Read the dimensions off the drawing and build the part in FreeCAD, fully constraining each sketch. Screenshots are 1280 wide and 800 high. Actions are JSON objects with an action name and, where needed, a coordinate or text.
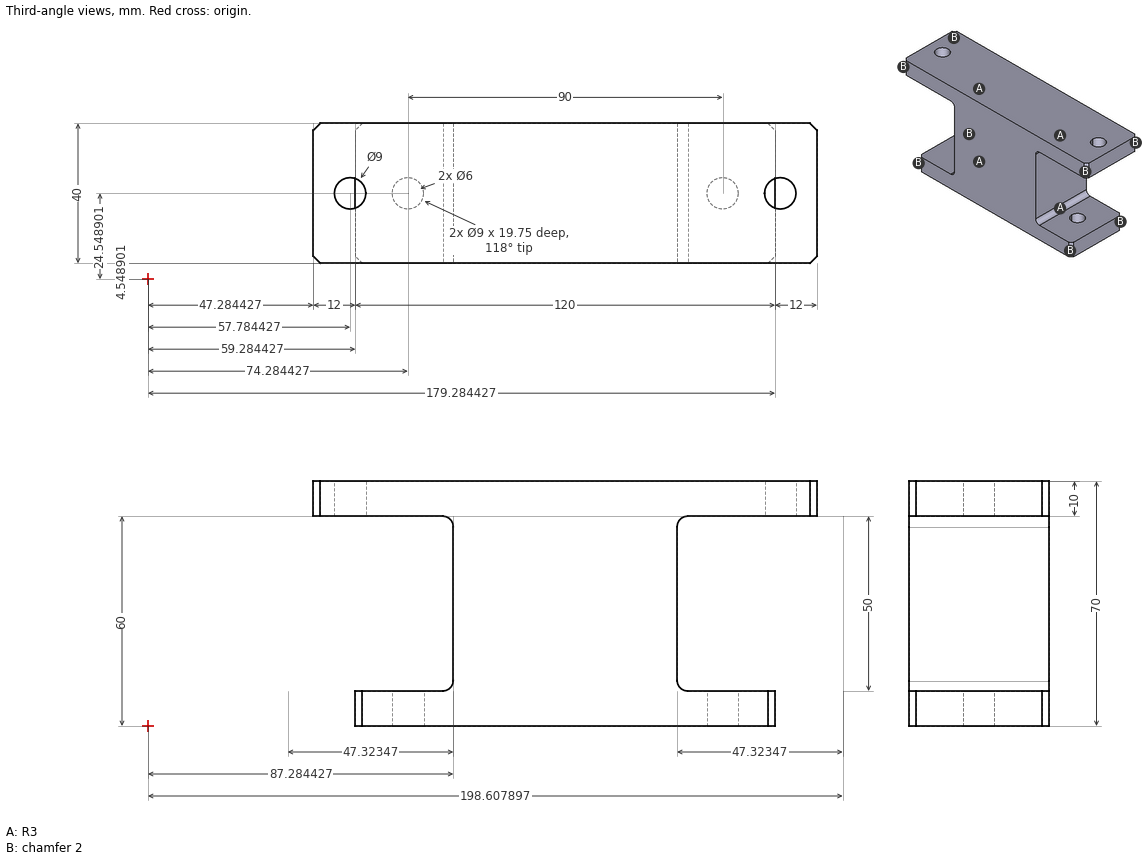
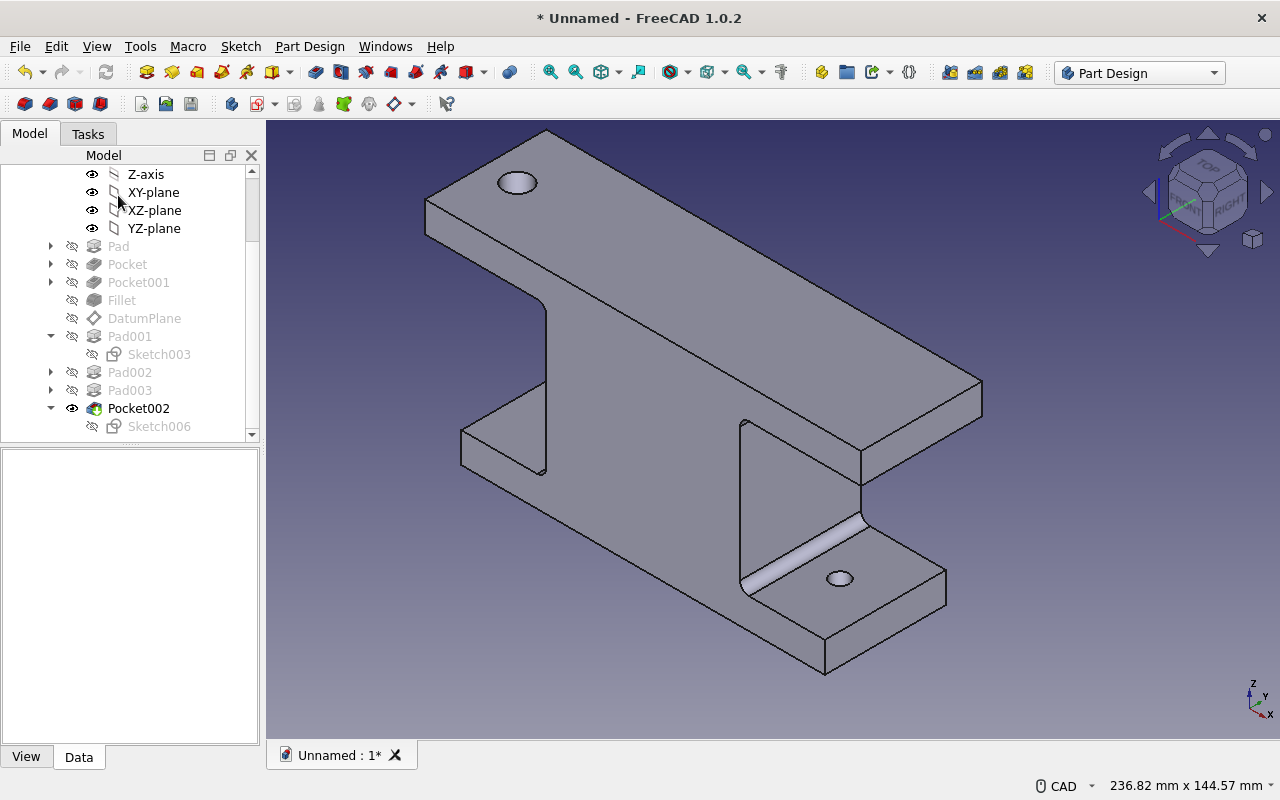
{"action": "scroll", "coordinate": [161, 296], "scroll_direction": "down", "scroll_amount": 3}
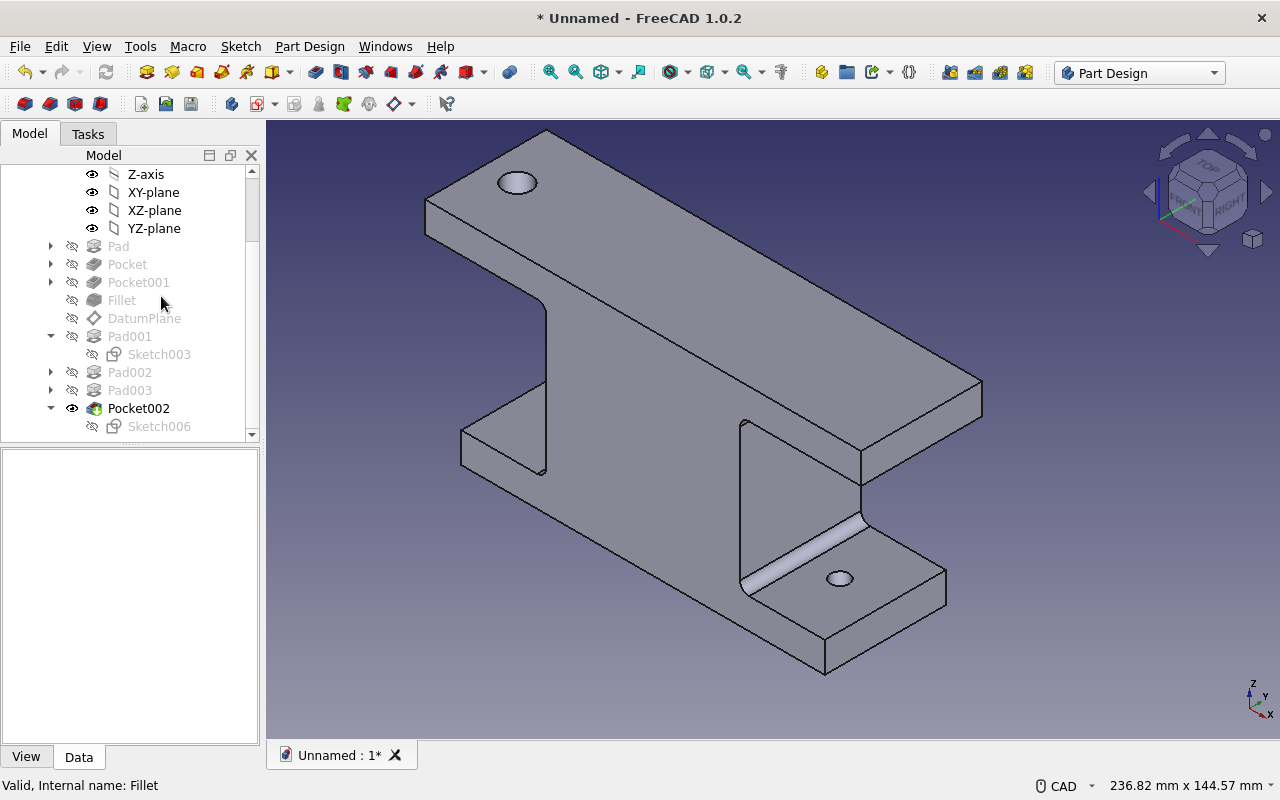
{"action": "scroll", "coordinate": [161, 296], "scroll_direction": "up", "scroll_amount": 15}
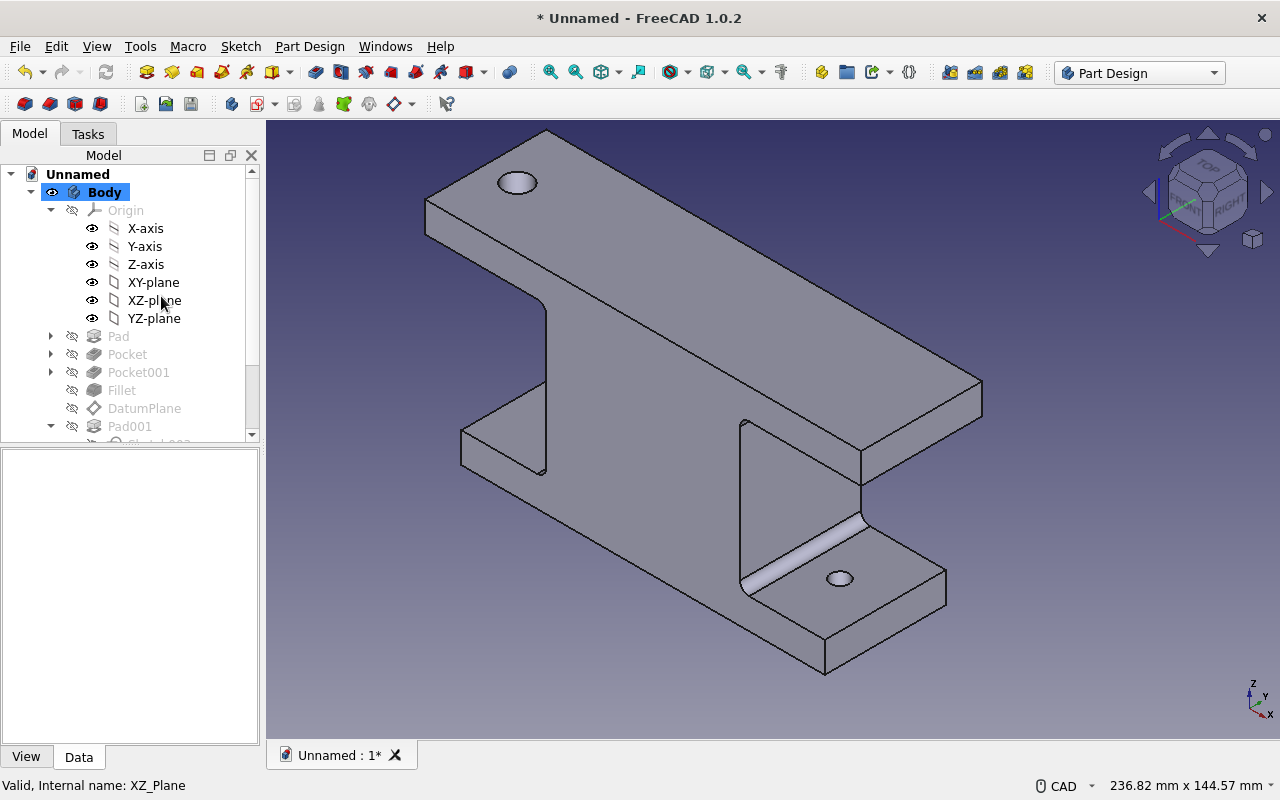
{"action": "left_click", "coordinate": [137, 318]}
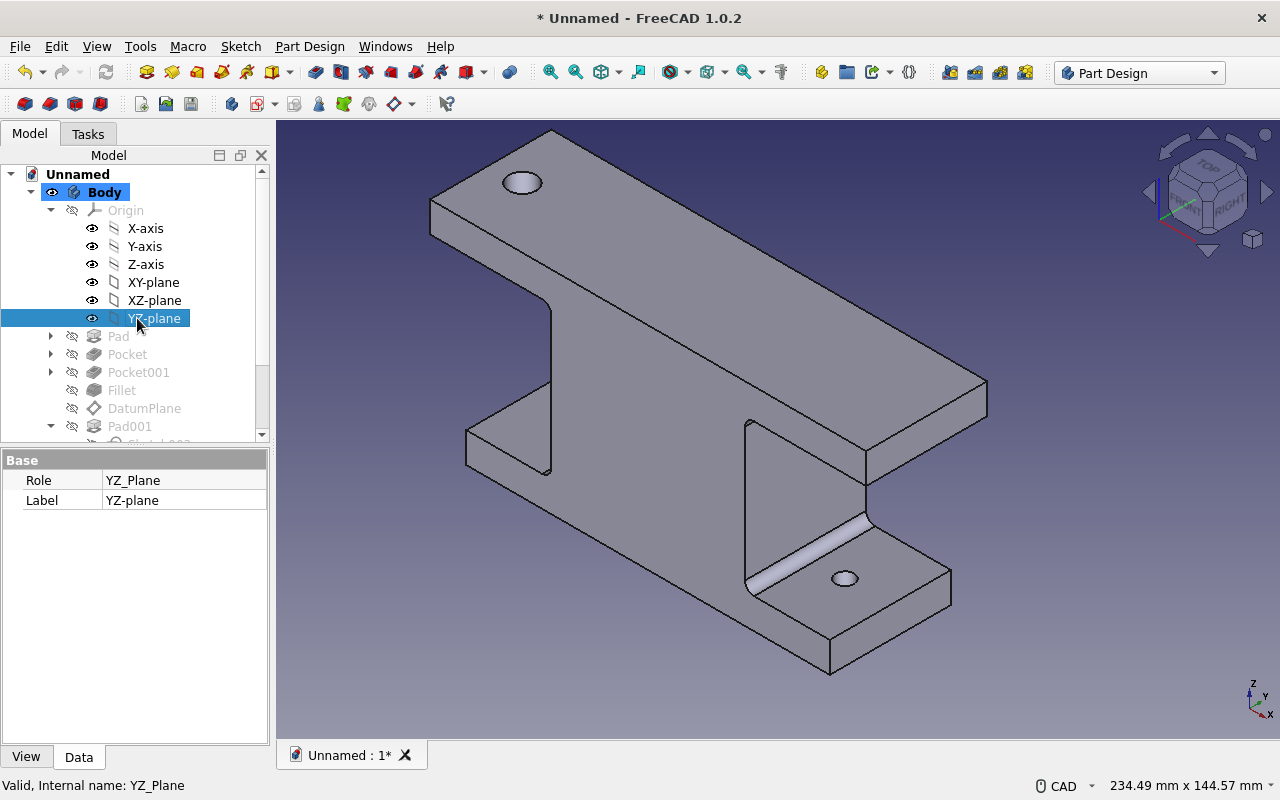
{"action": "left_click", "coordinate": [394, 104]}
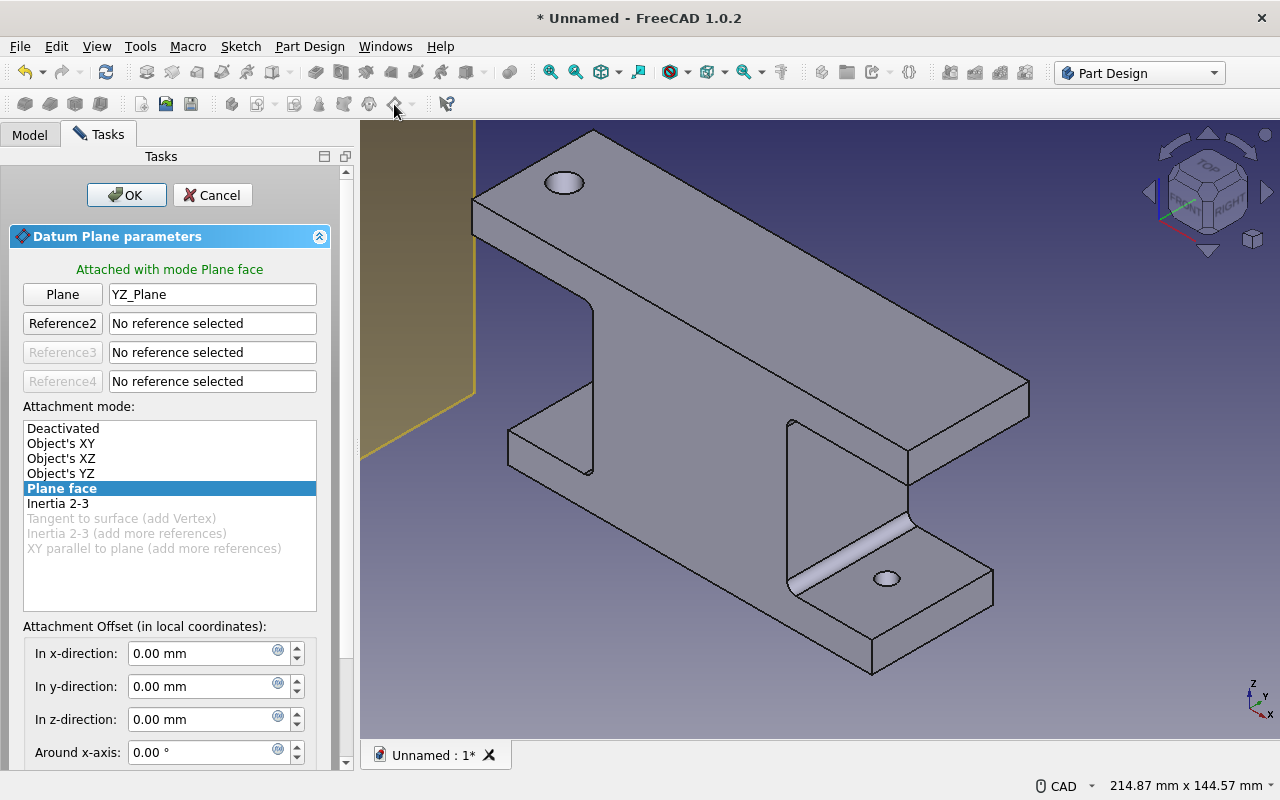
{"action": "triple_click", "coordinate": [210, 720]}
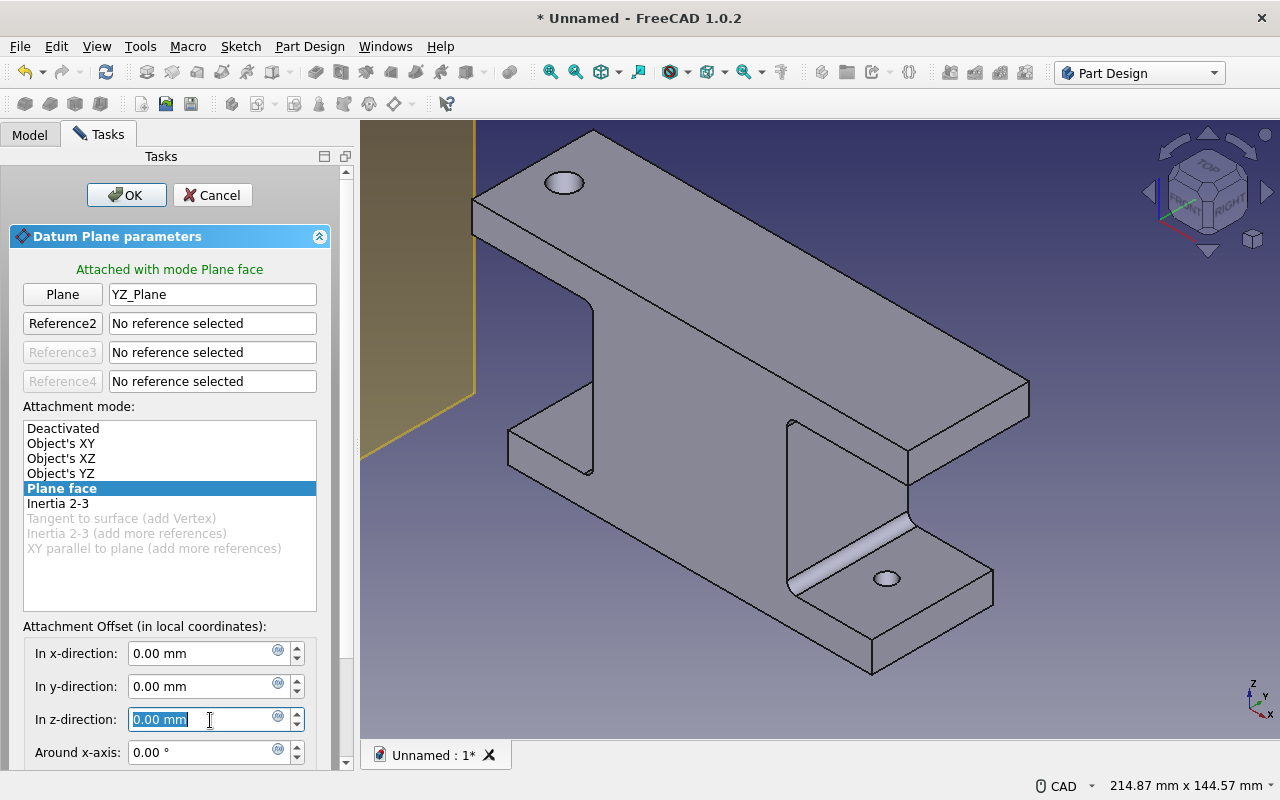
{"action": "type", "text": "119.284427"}
{"action": "key", "text": "Tab"}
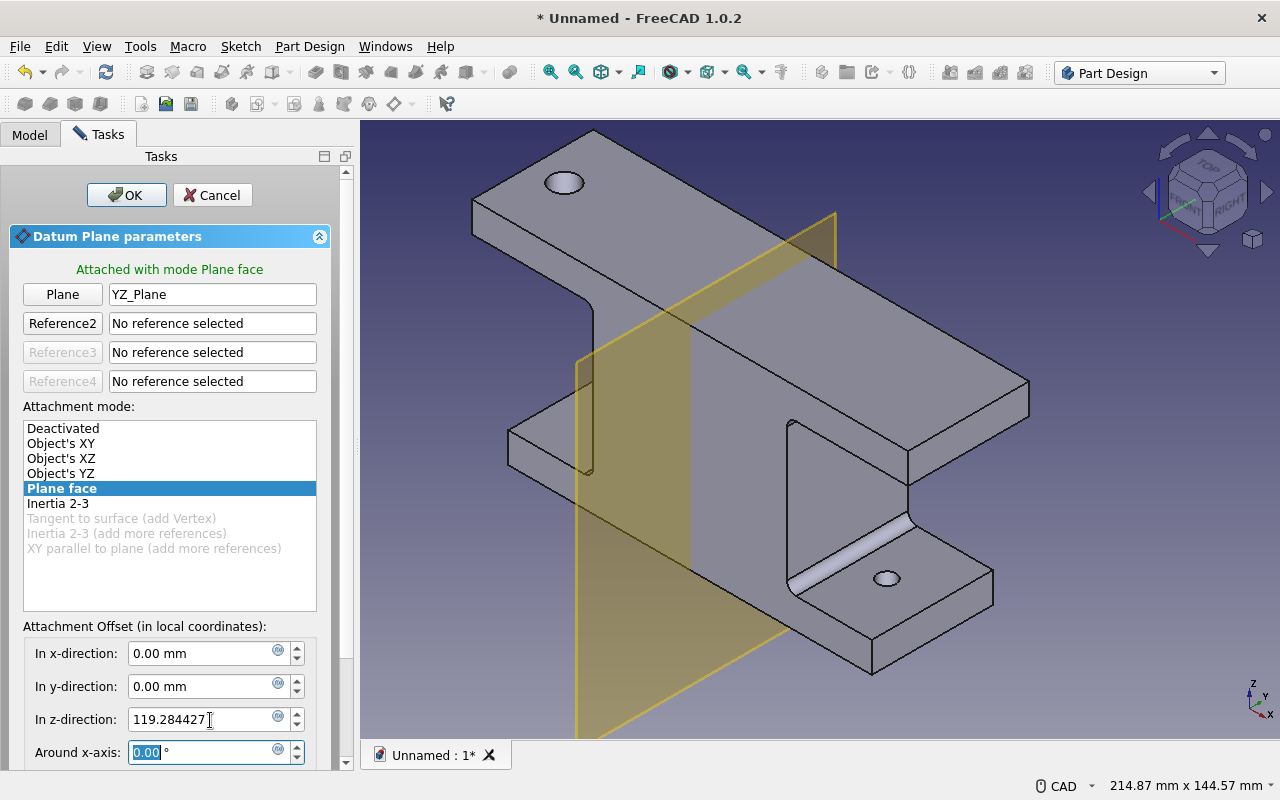
{"action": "left_click", "coordinate": [127, 195]}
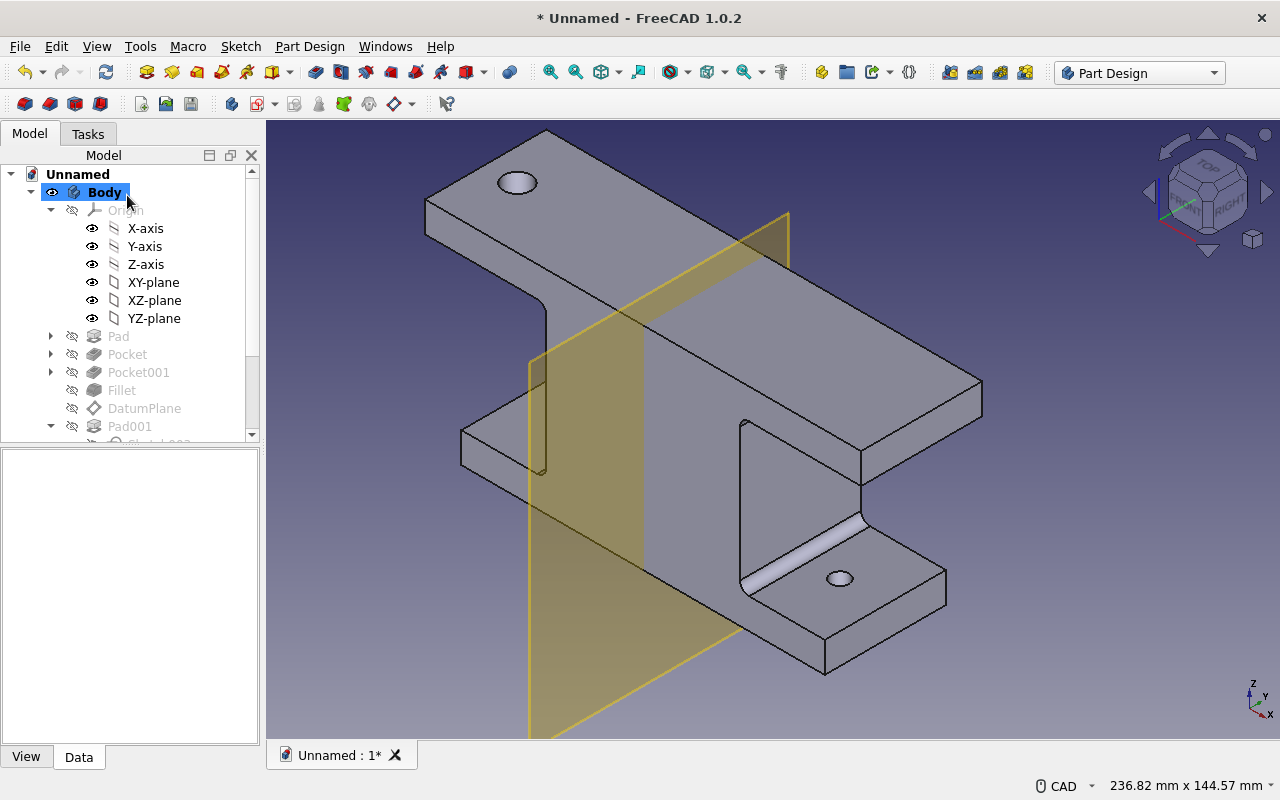
{"action": "scroll", "coordinate": [101, 296], "scroll_direction": "down", "scroll_amount": 3}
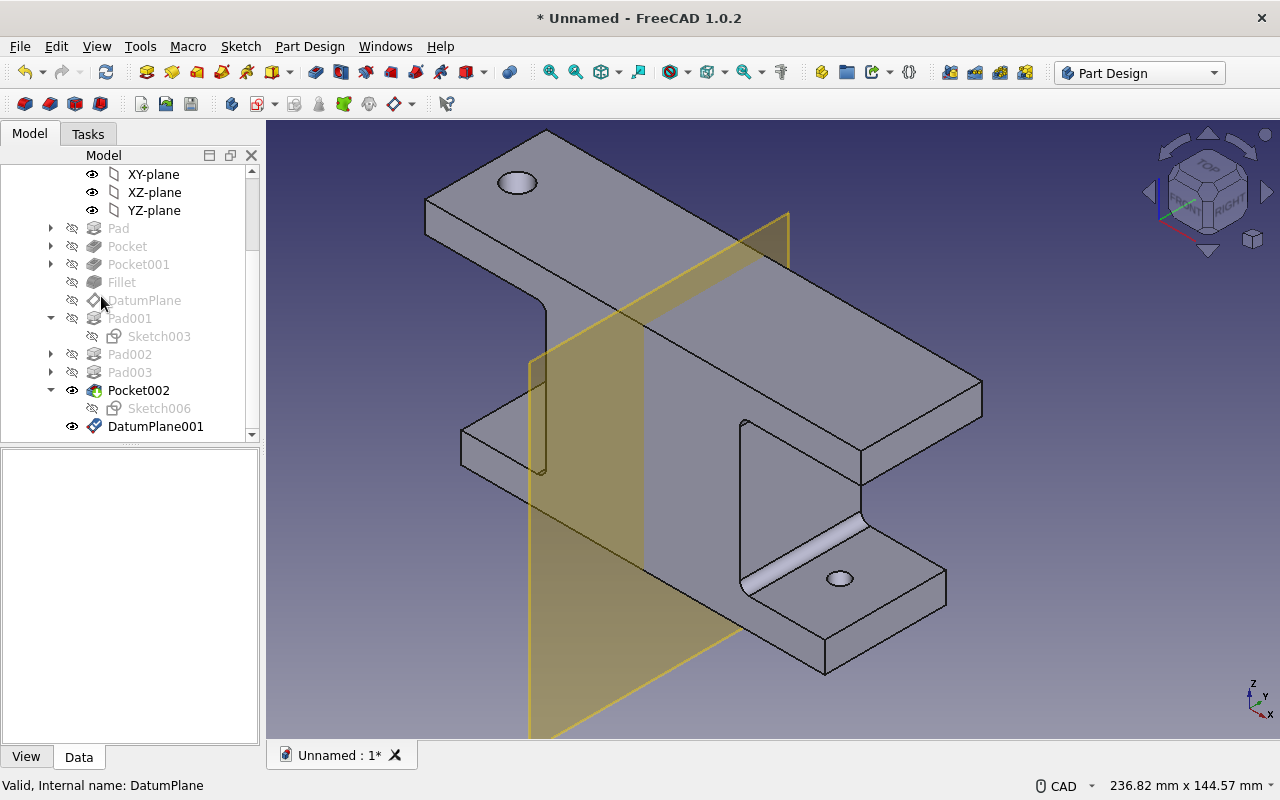
{"action": "left_click", "coordinate": [117, 390]}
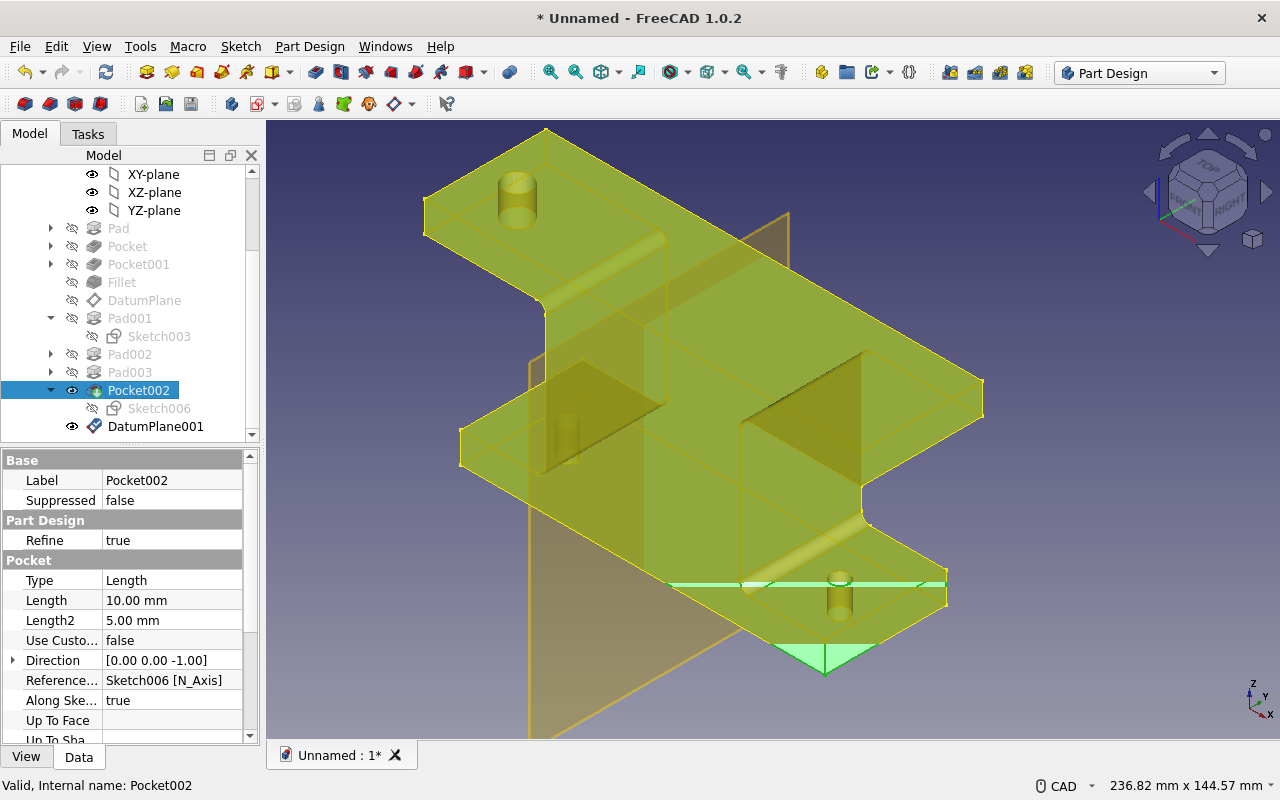
{"action": "left_click", "coordinate": [950, 72]}